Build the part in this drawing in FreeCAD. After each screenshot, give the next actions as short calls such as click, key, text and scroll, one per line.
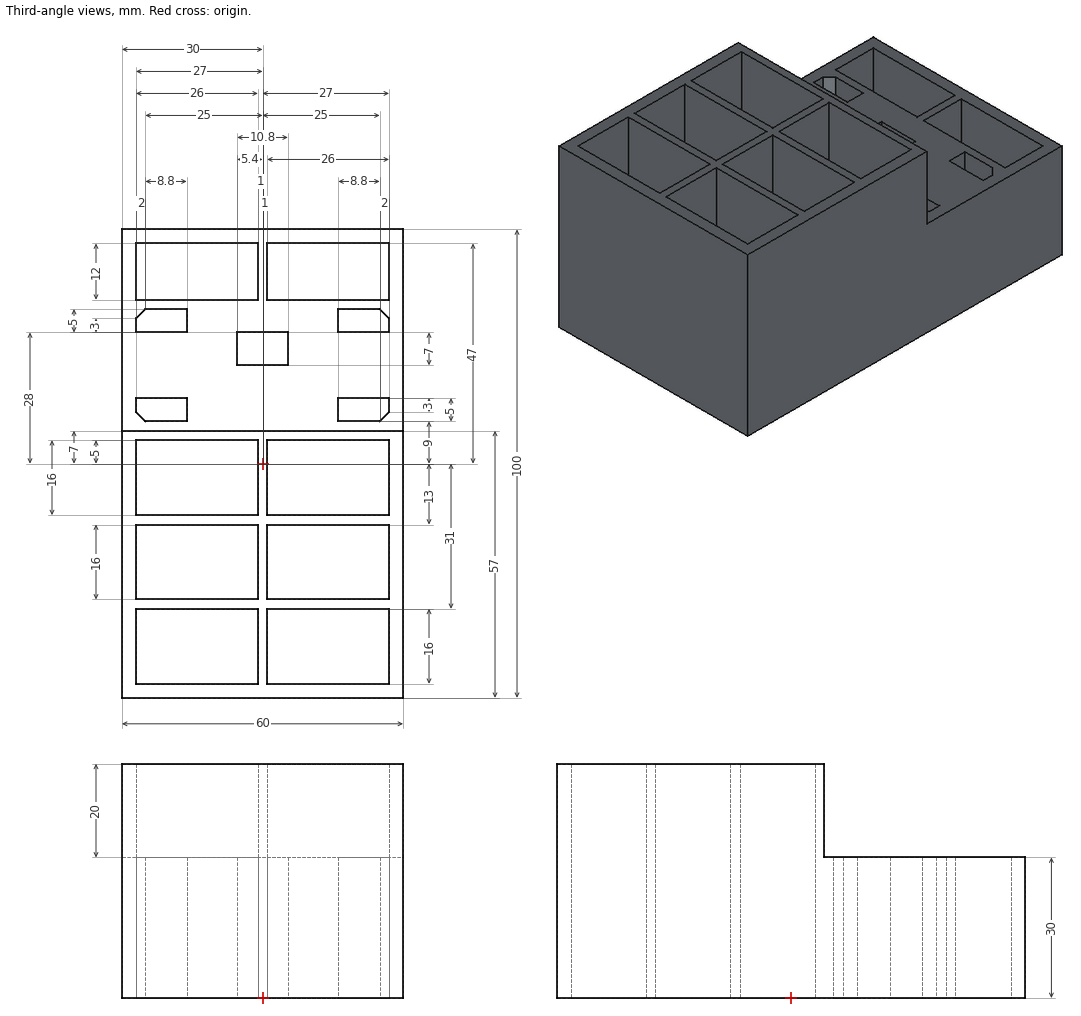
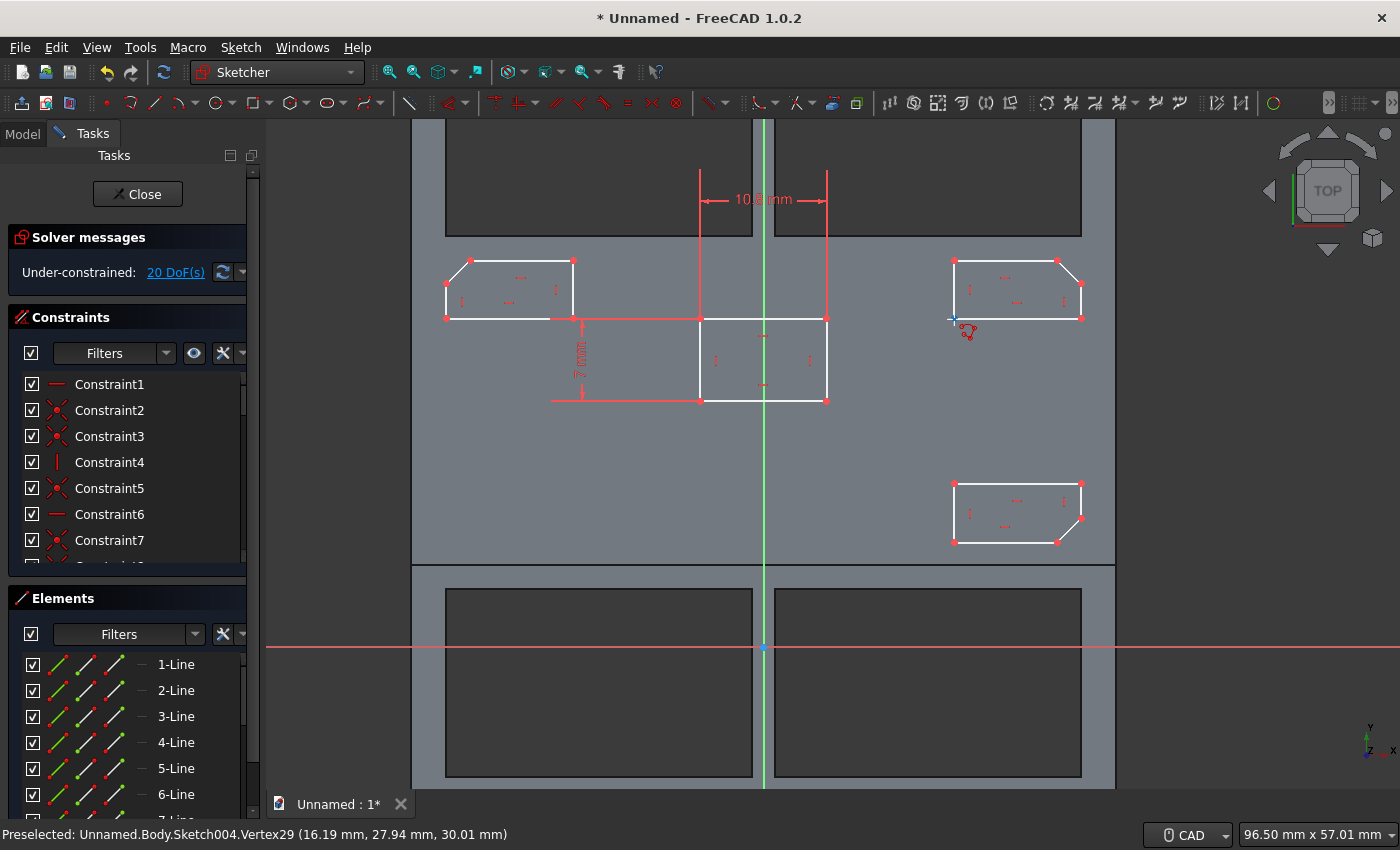
click(573, 542)
click(573, 483)
click(446, 483)
click(446, 518)
click(470, 542)
click(573, 543)
key(Escape)
key(Escape)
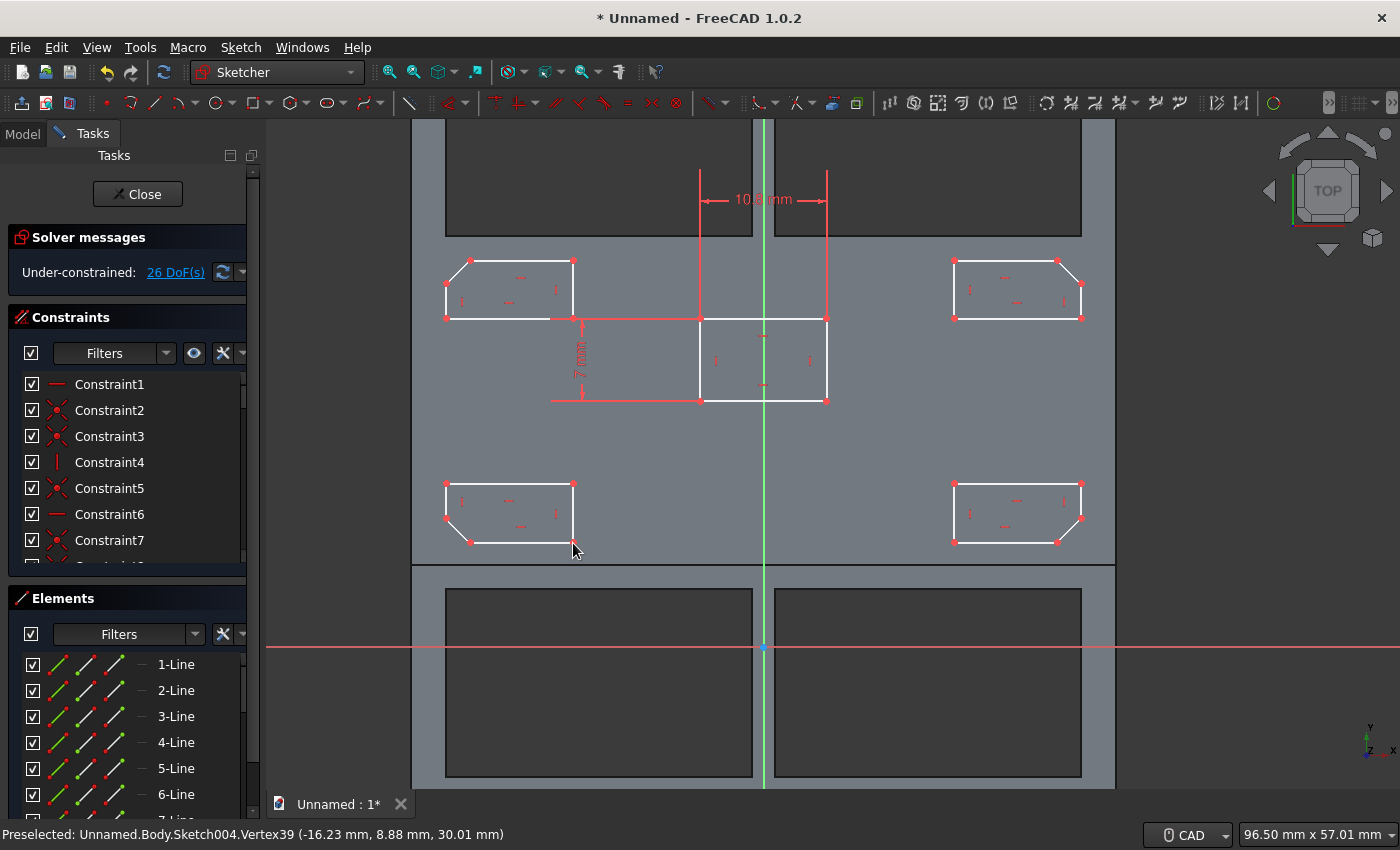
key(d)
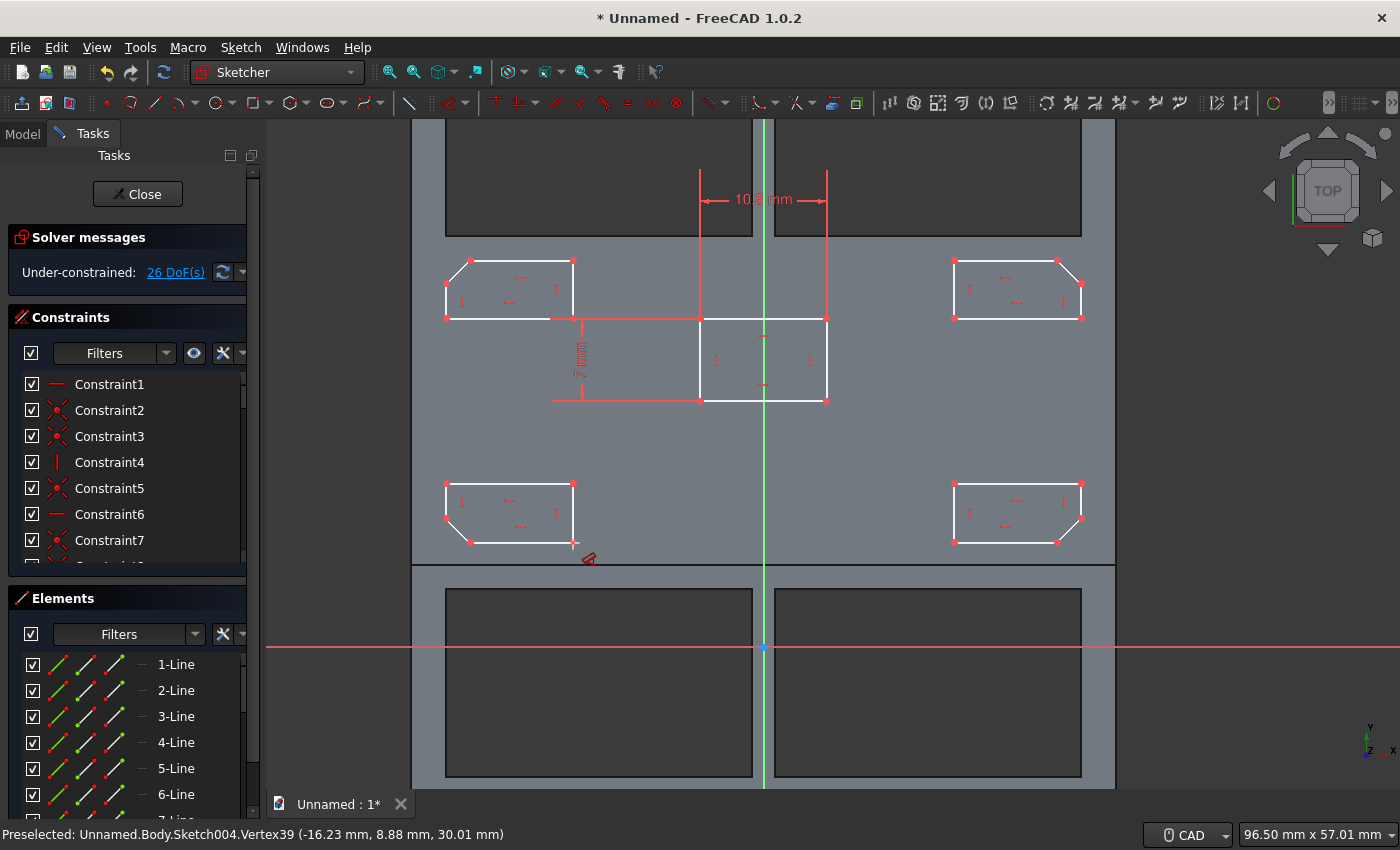
scroll(1081, 509, up, 2)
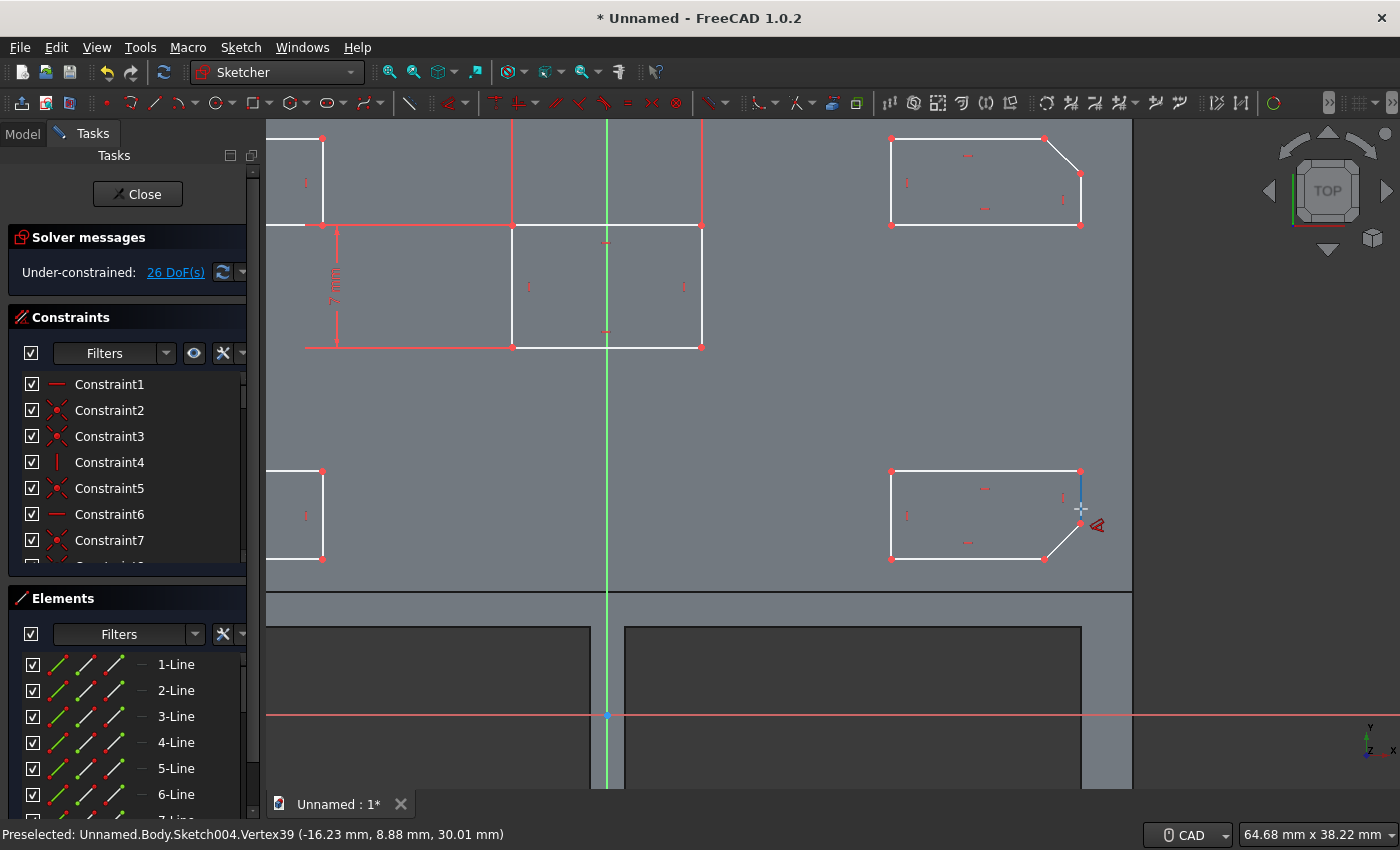
click(1081, 508)
click(1115, 498)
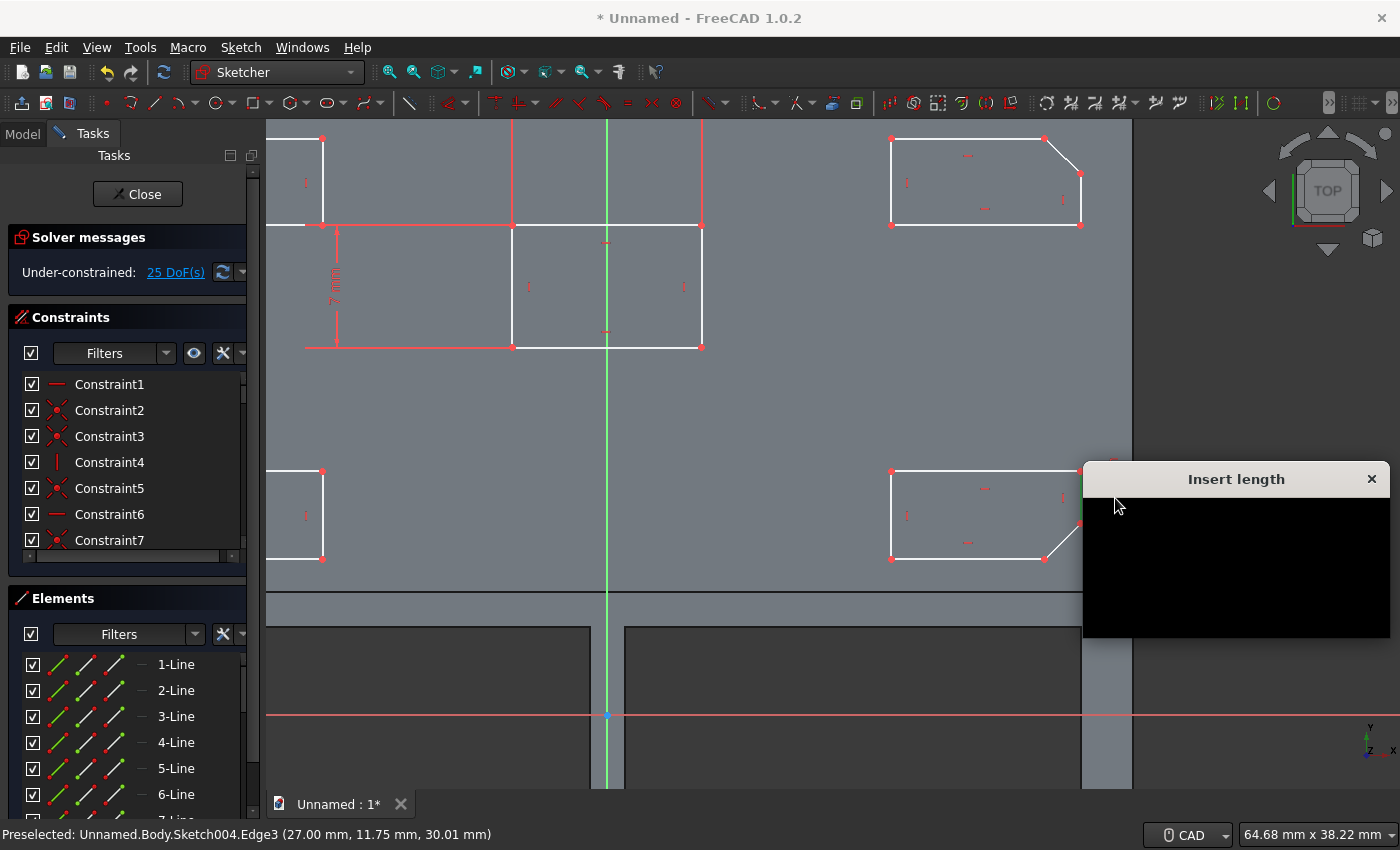
text(3)
key(Return)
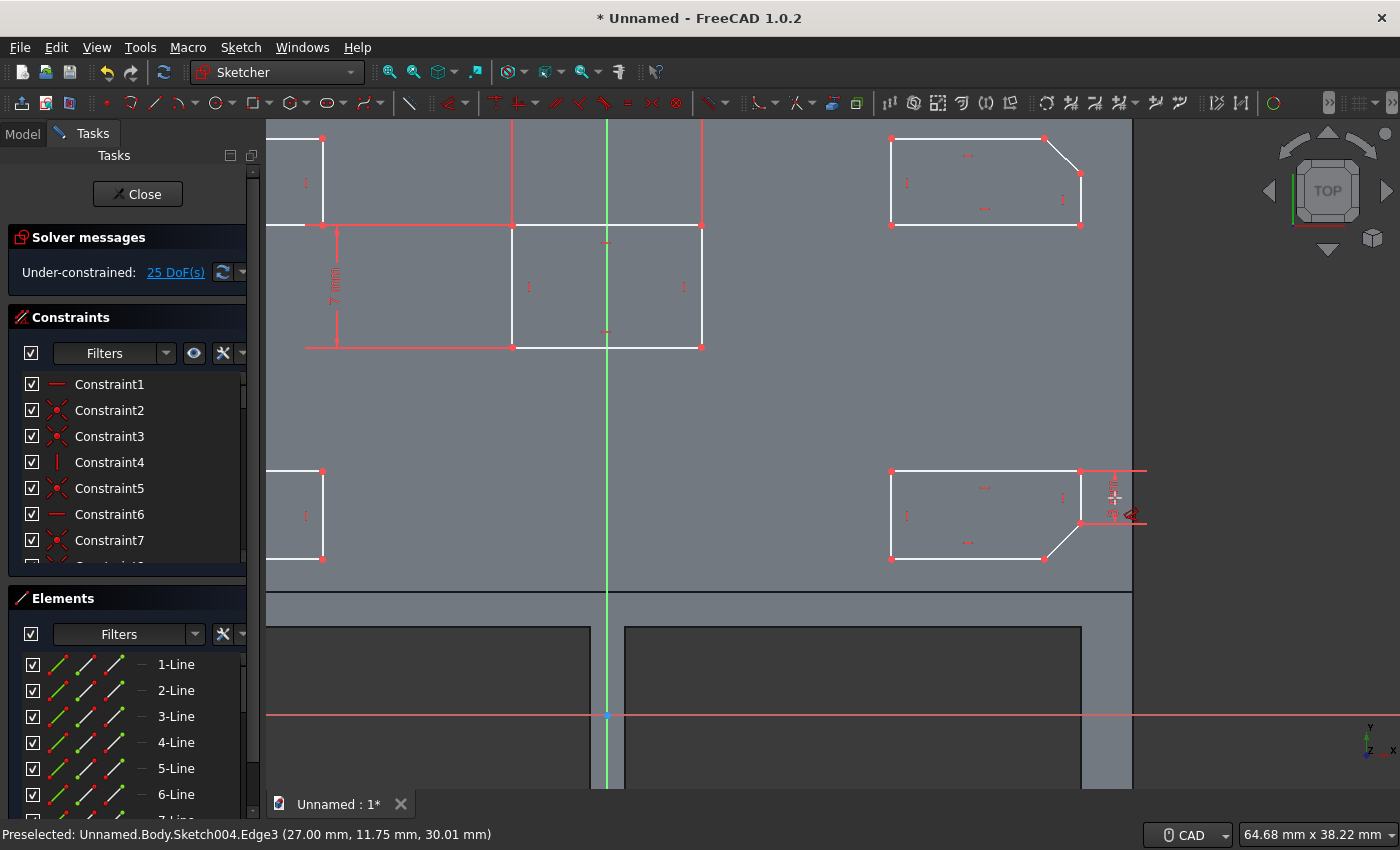
click(891, 498)
click(925, 515)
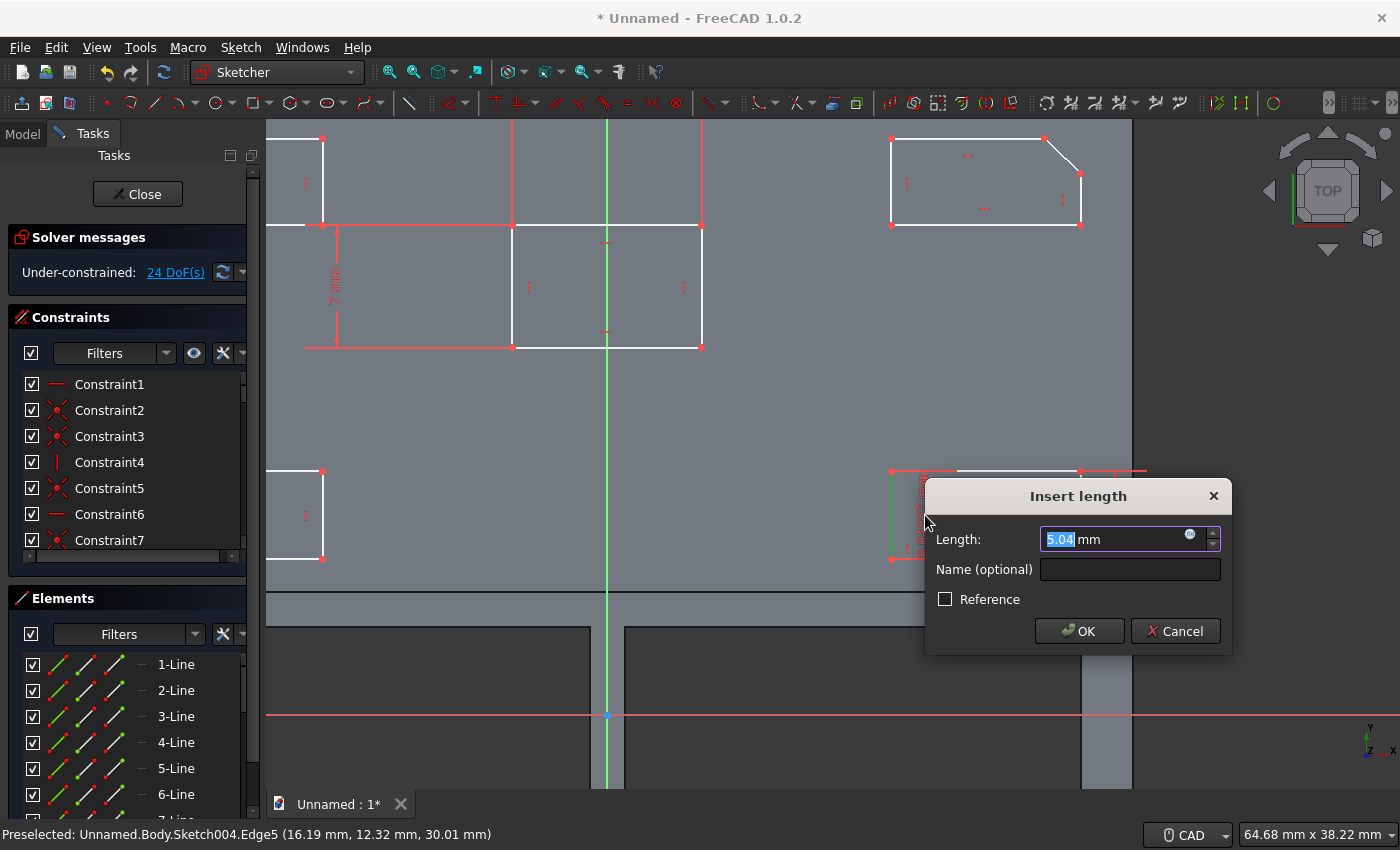
text(5)
key(Return)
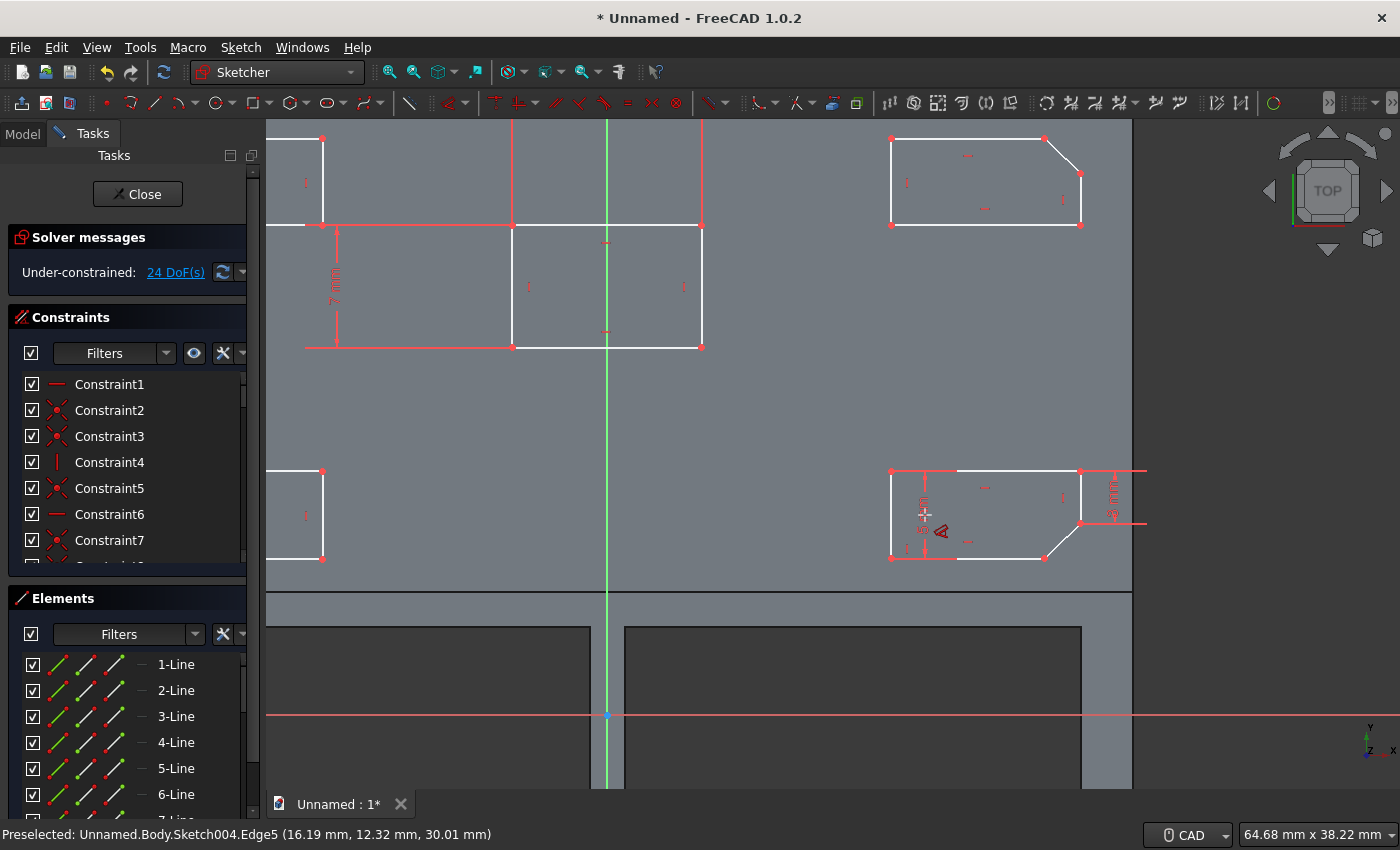
click(323, 199)
click(357, 186)